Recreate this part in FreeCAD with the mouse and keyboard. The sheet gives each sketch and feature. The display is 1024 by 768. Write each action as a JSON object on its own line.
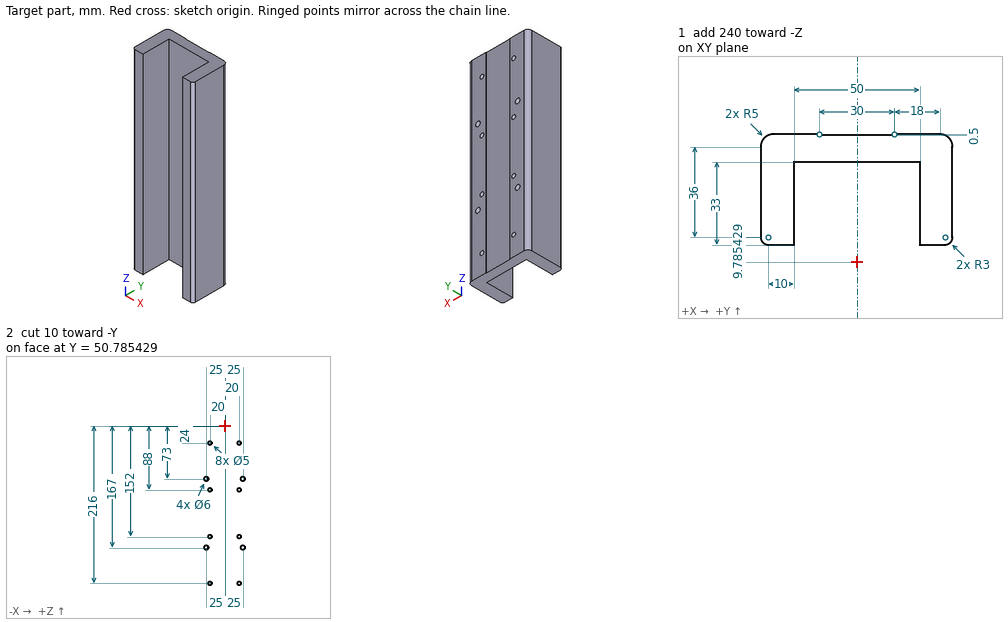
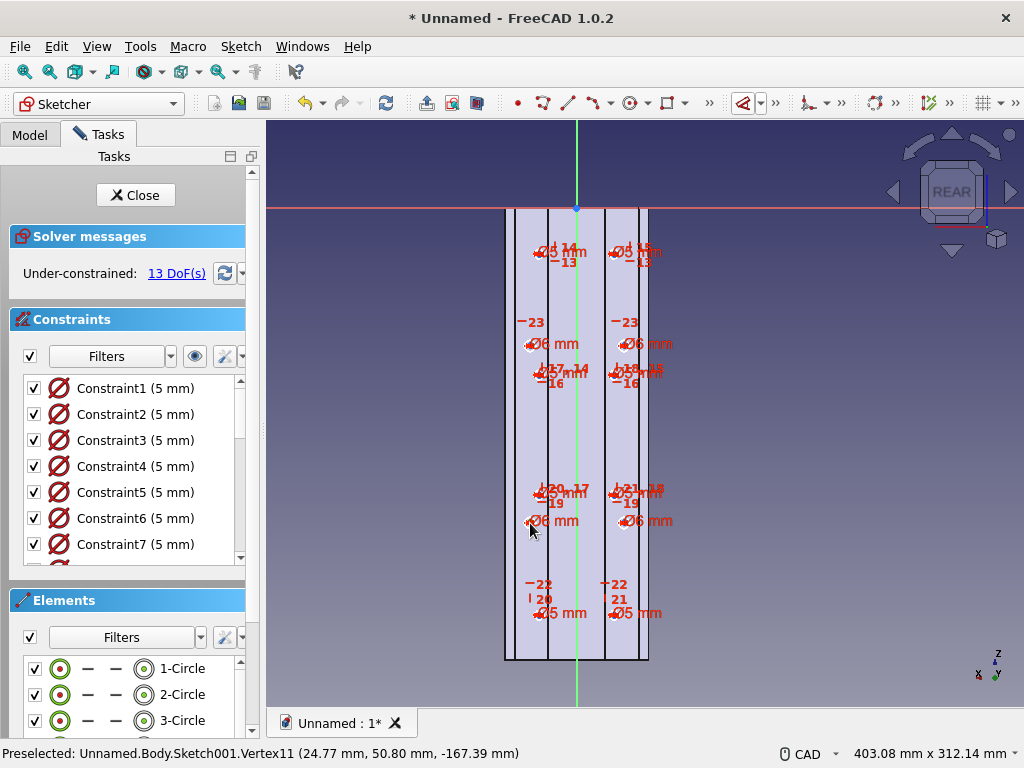
{"action": "left_click", "coordinate": [624, 523]}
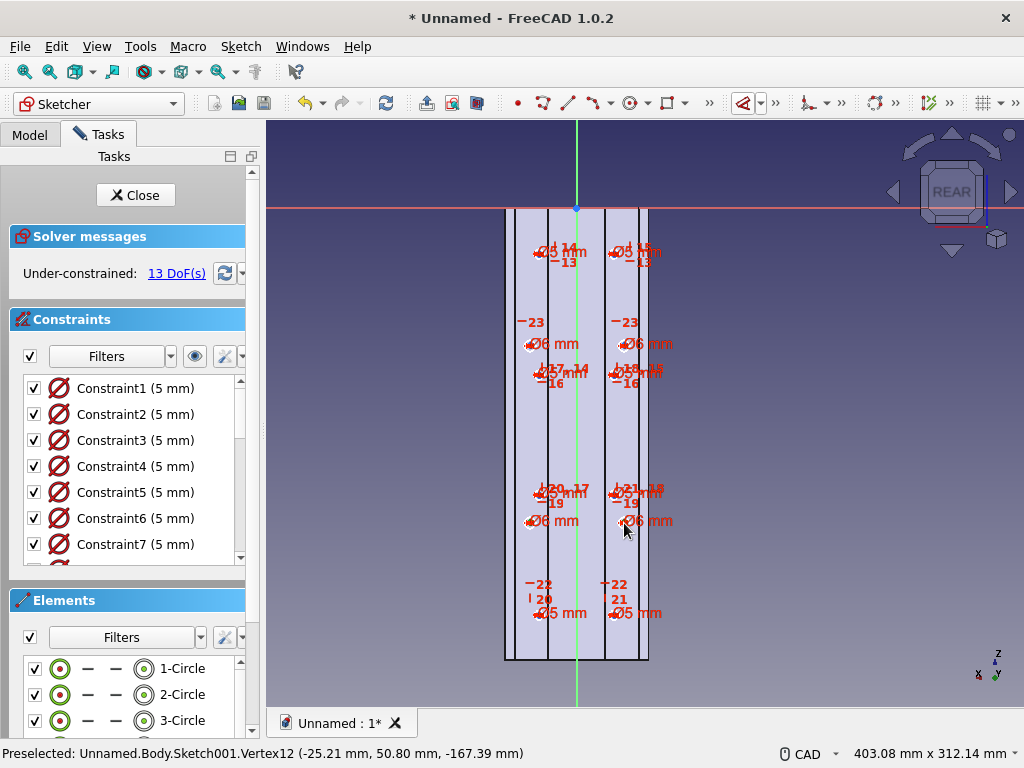
{"action": "key", "text": "h"}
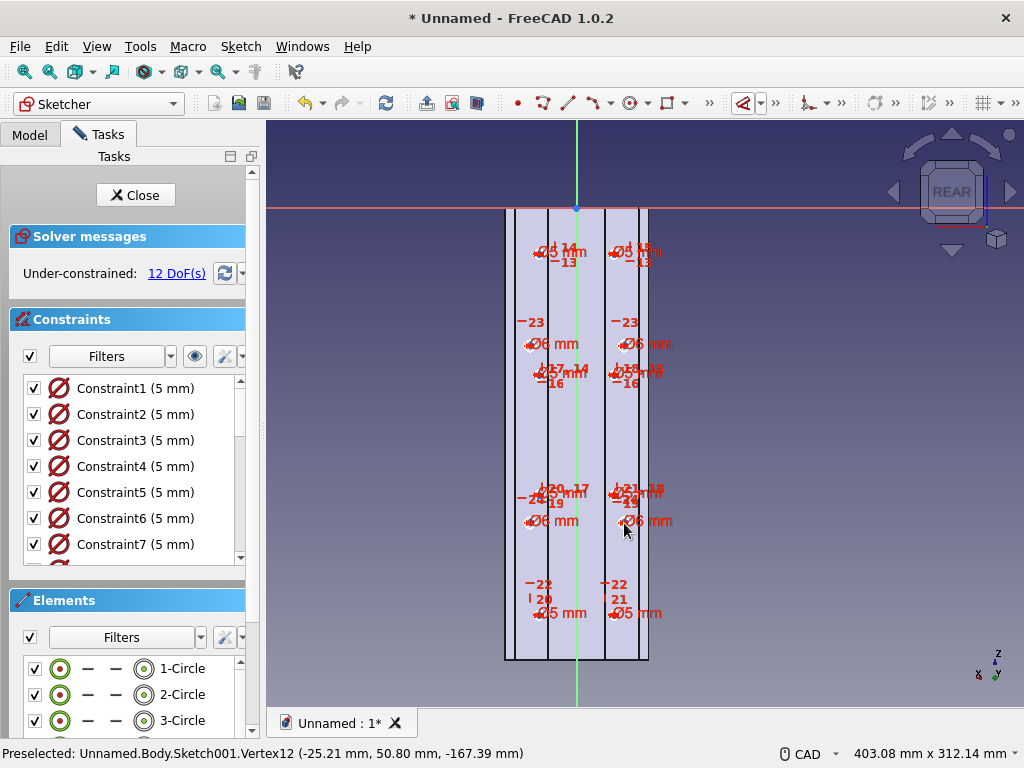
{"action": "left_click", "coordinate": [539, 254]}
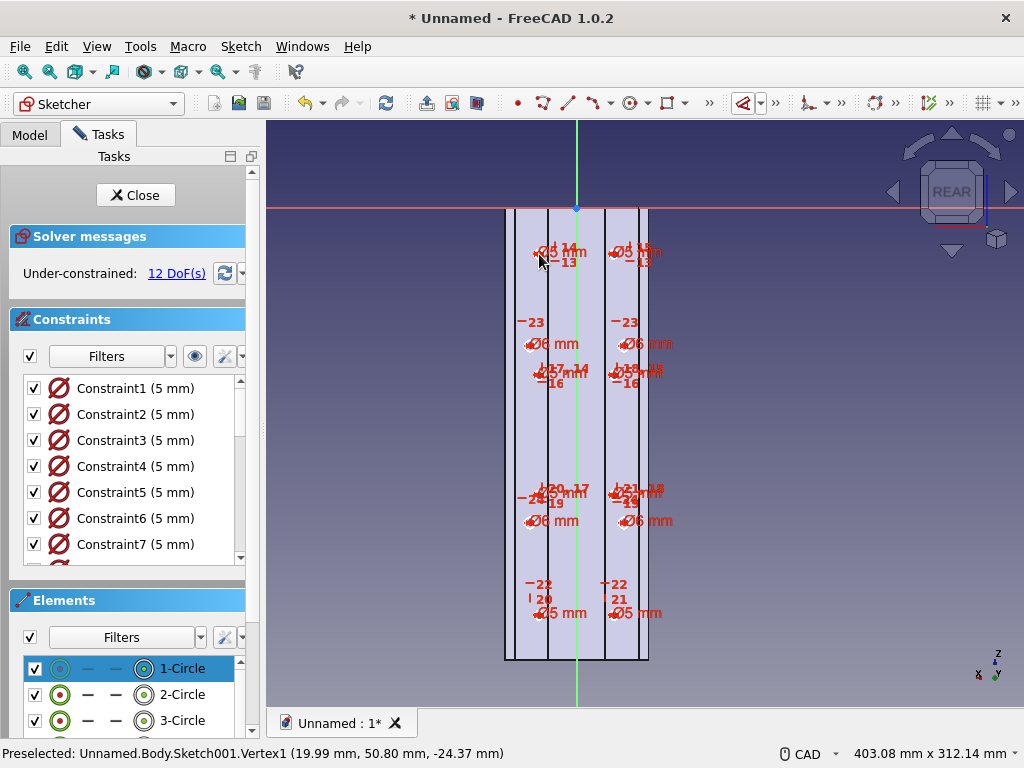
{"action": "left_click", "coordinate": [760, 104]}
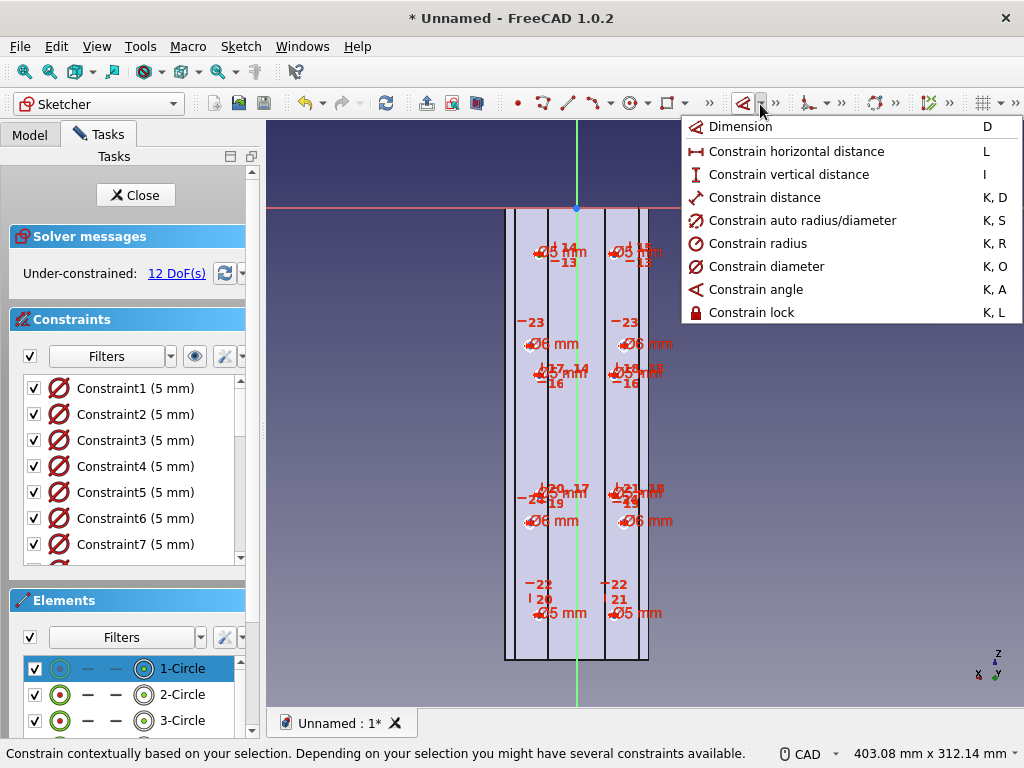
{"action": "left_click", "coordinate": [852, 152]}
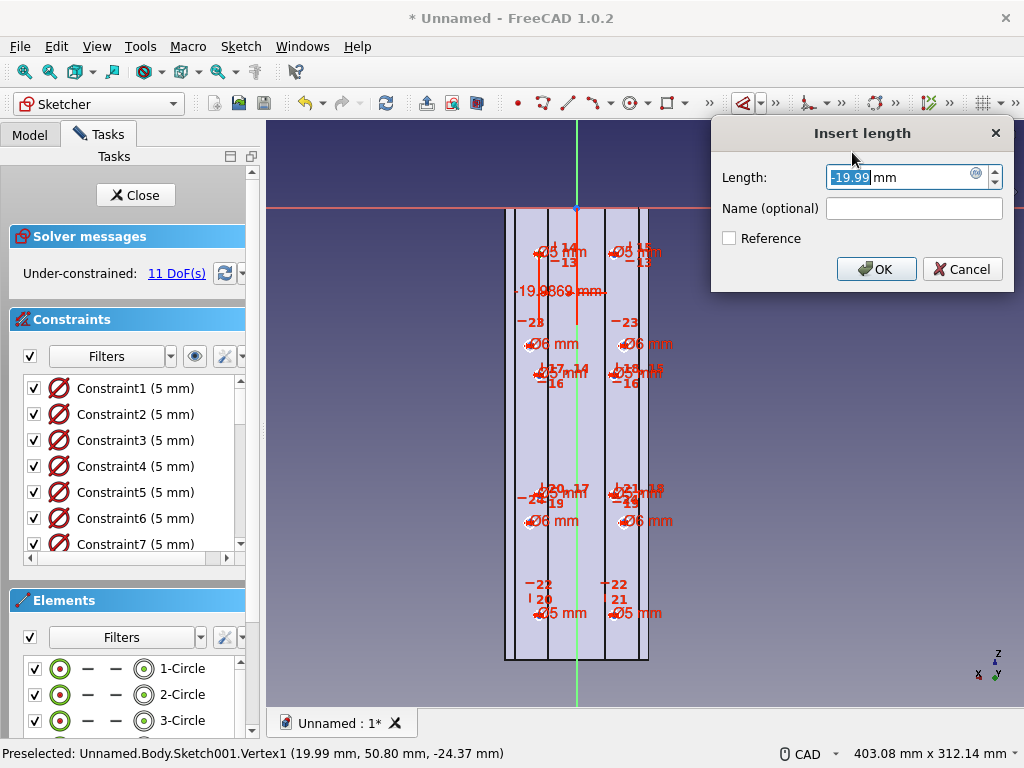
{"action": "type", "text": "-20"}
{"action": "key", "text": "Return"}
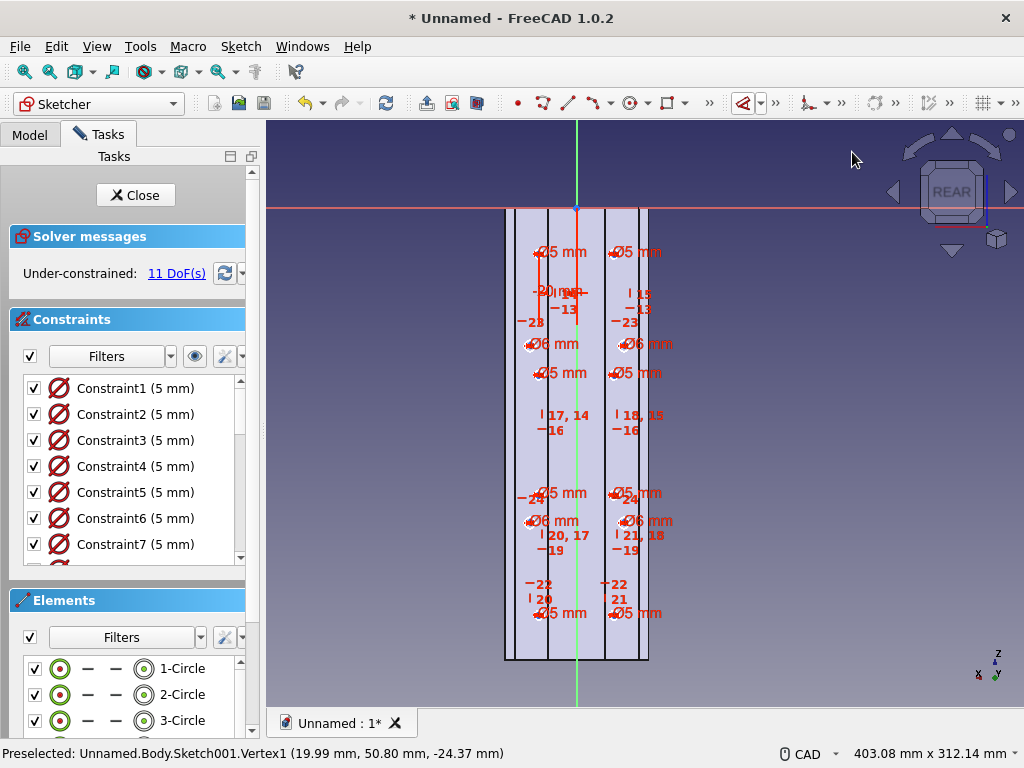
{"action": "left_click", "coordinate": [539, 254]}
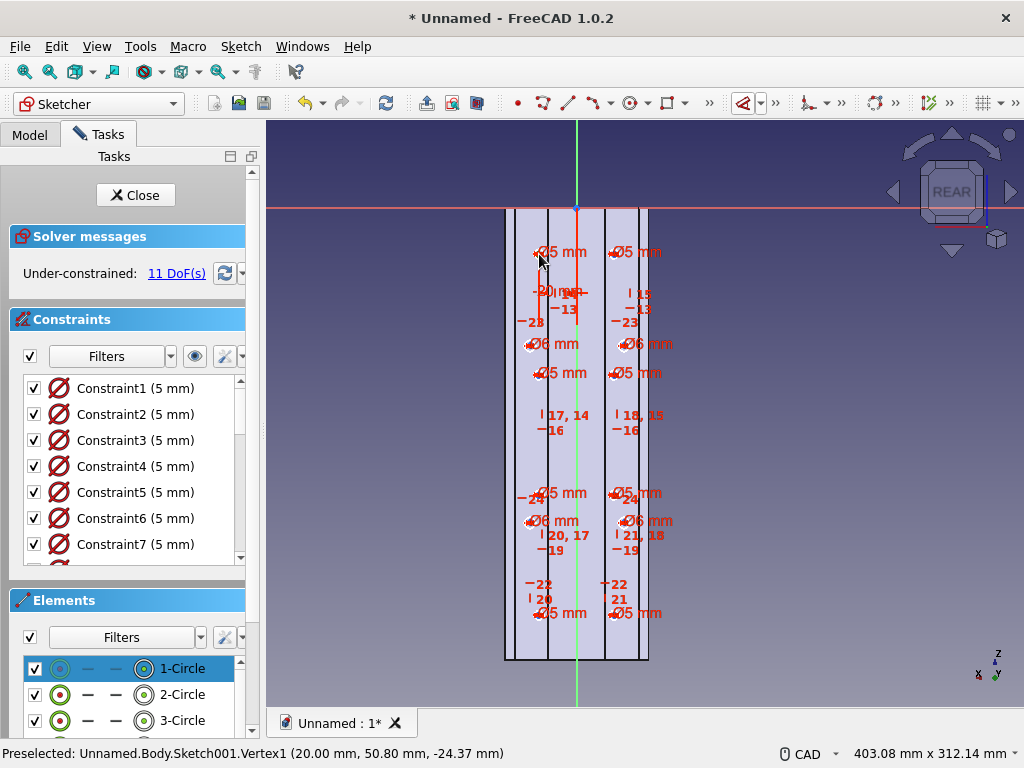
{"action": "left_click", "coordinate": [760, 104]}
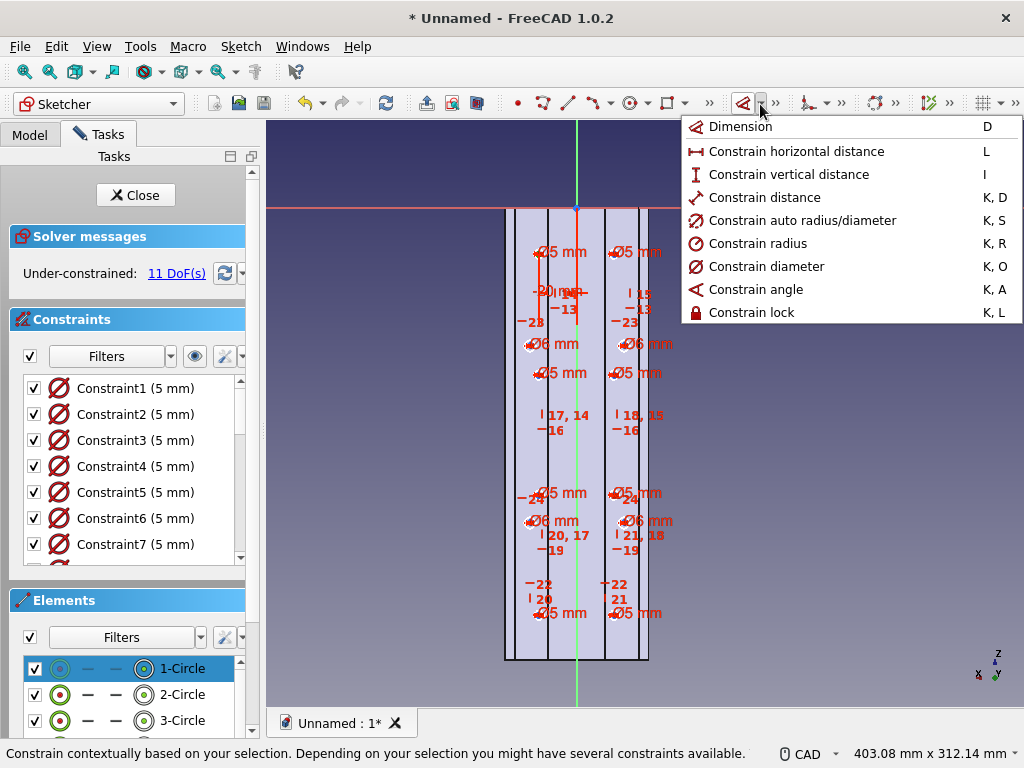
{"action": "left_click", "coordinate": [852, 174]}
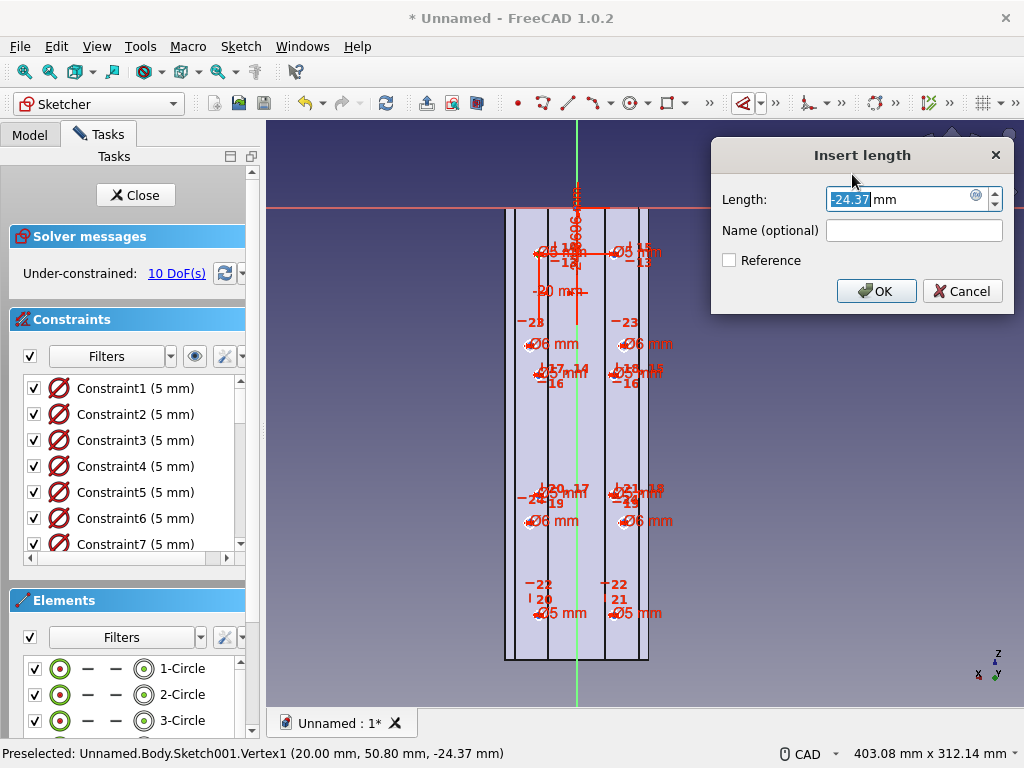
{"action": "type", "text": "-24"}
{"action": "key", "text": "Return"}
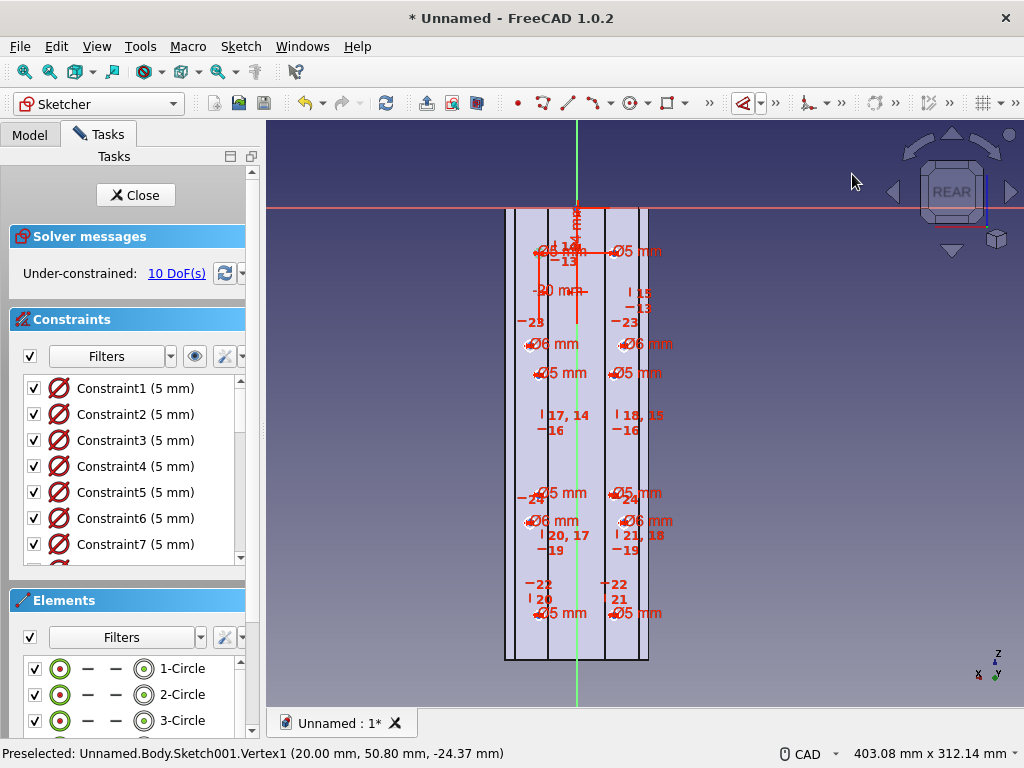
{"action": "left_click", "coordinate": [614, 253]}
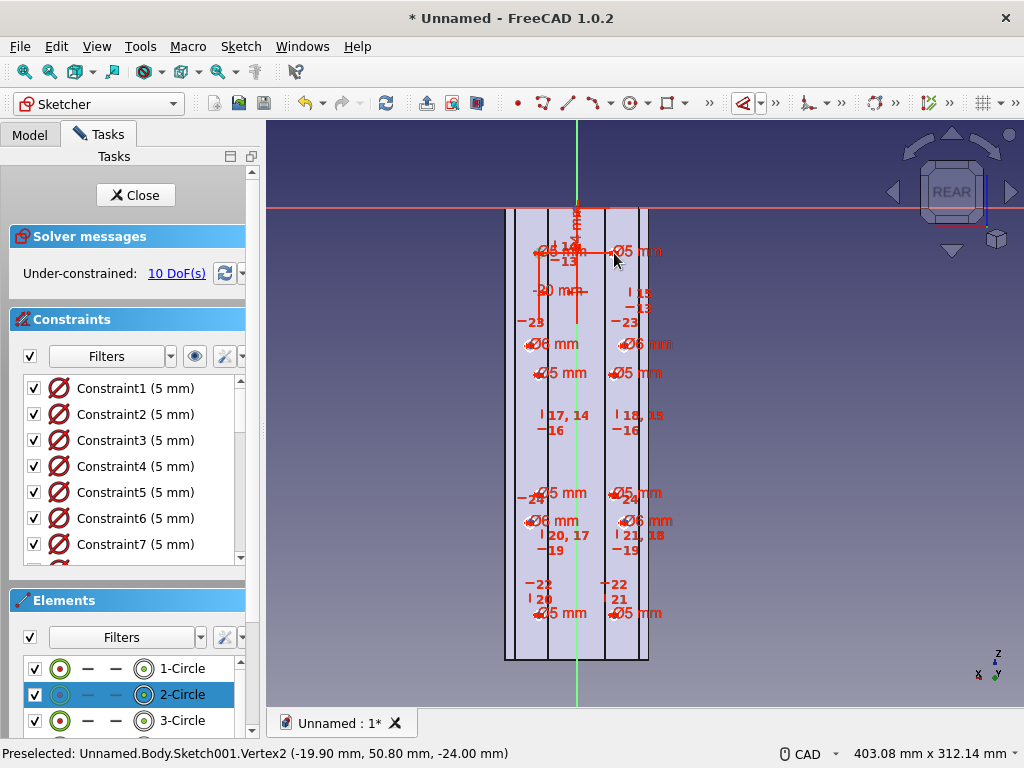
{"action": "key", "text": "l"}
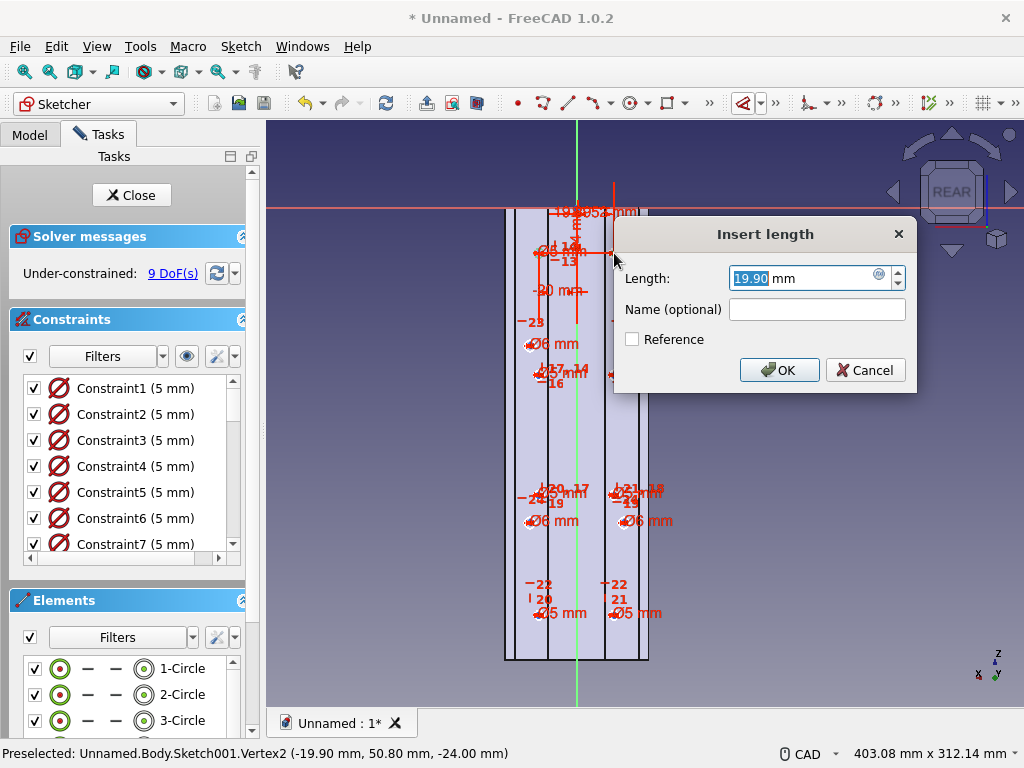
{"action": "type", "text": "20"}
{"action": "key", "text": "Return"}